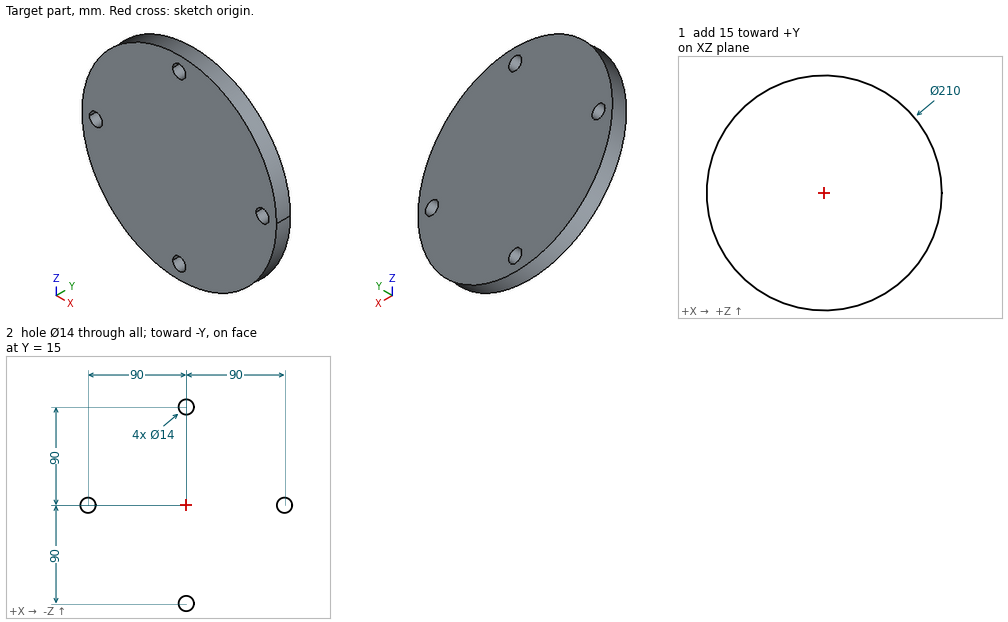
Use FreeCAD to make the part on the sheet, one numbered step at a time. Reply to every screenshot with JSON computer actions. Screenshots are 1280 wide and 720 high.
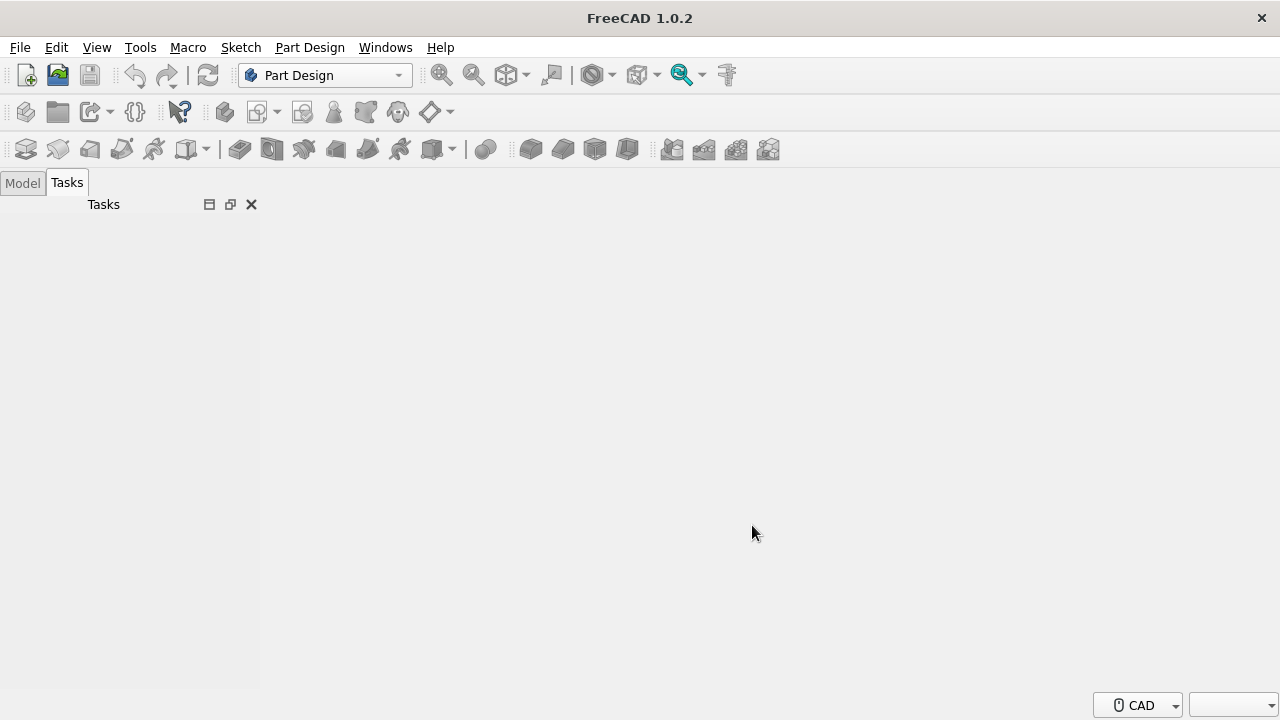
{"action": "key", "text": "ctrl+n"}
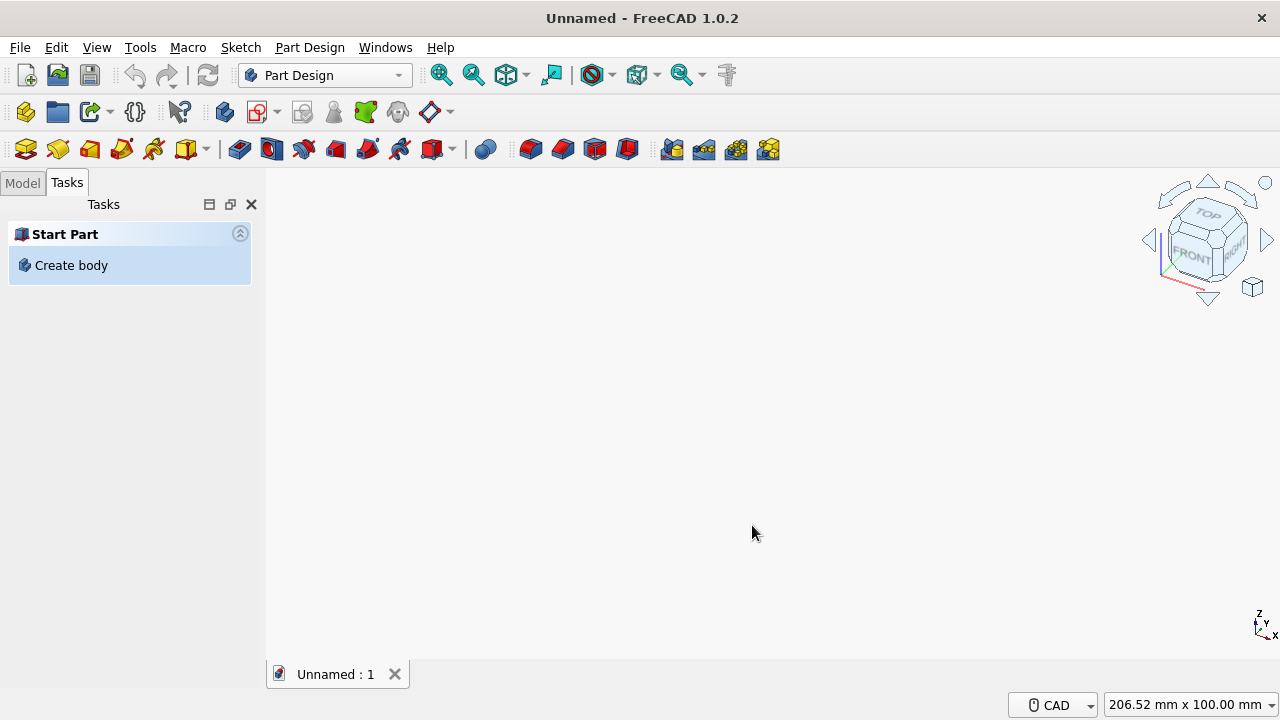
{"action": "left_click", "coordinate": [258, 112]}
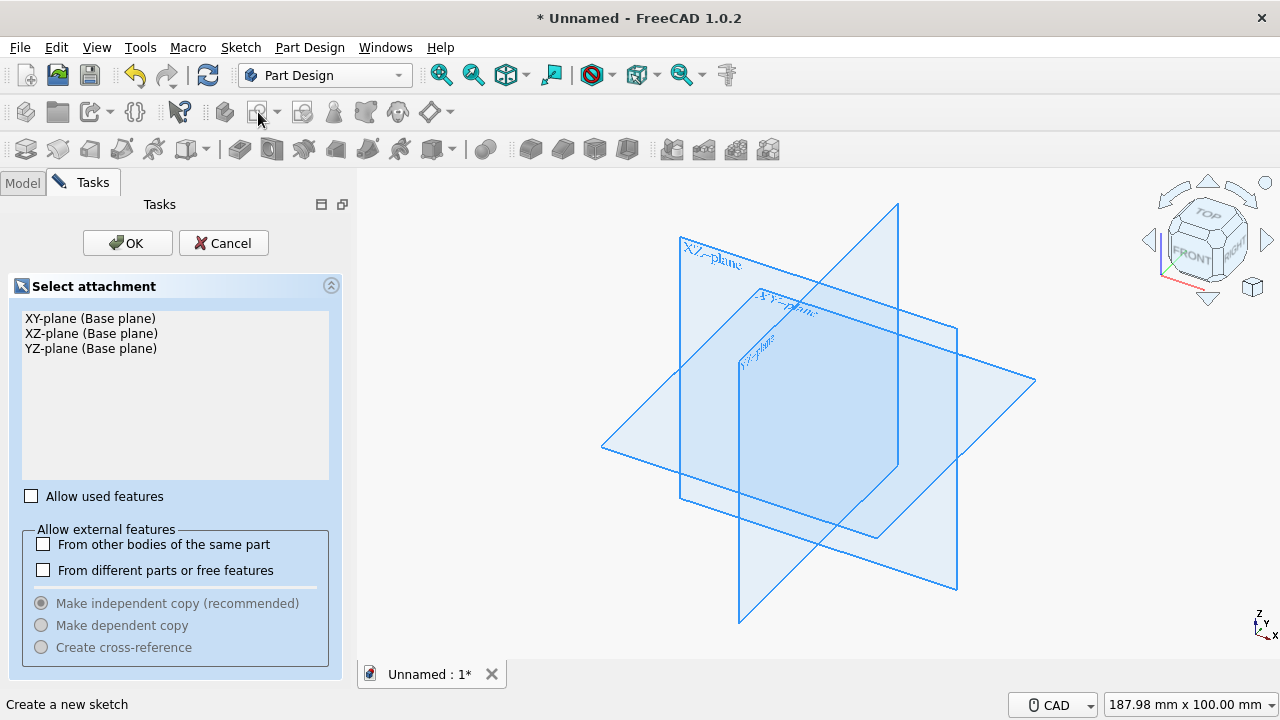
{"action": "left_click", "coordinate": [82, 334]}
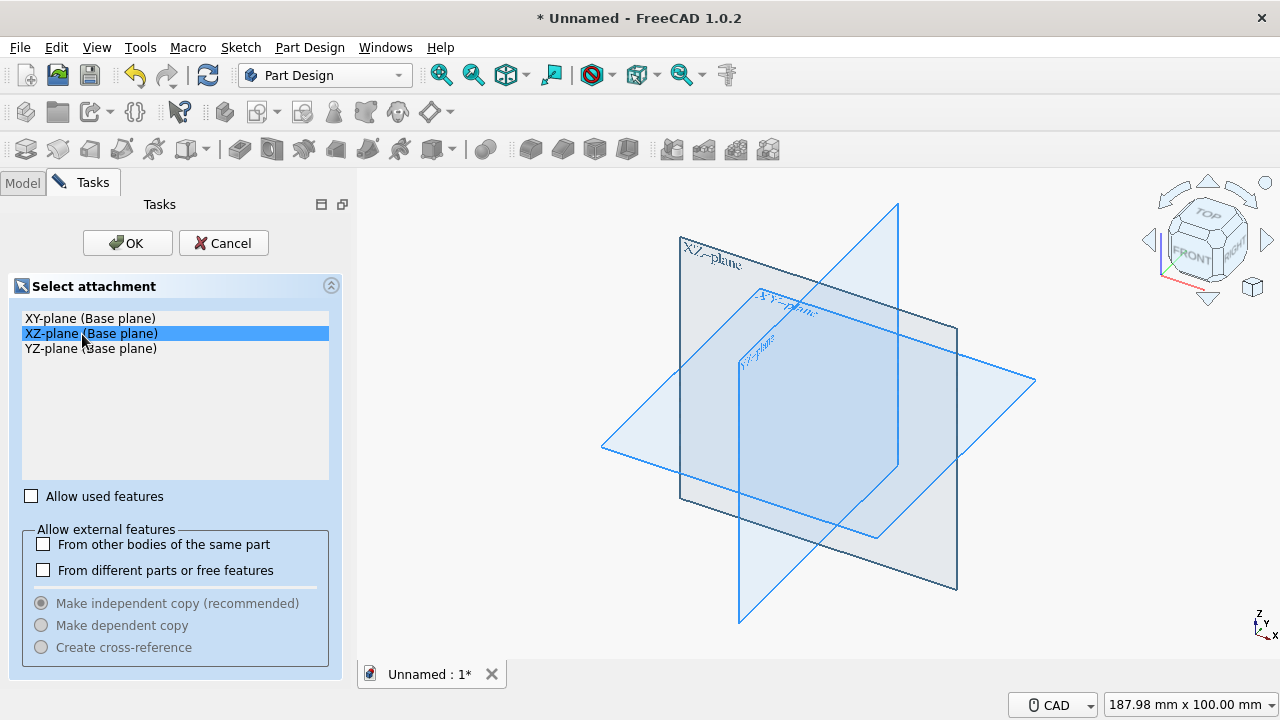
{"action": "left_click", "coordinate": [128, 243]}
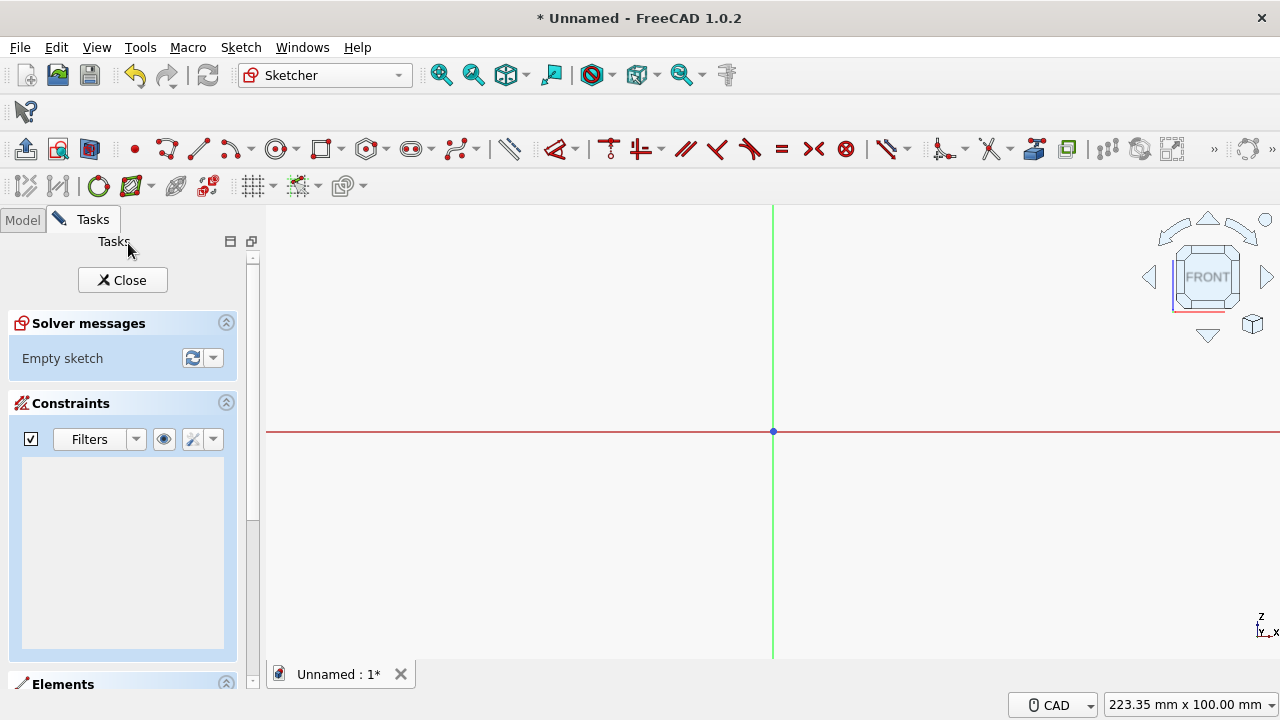
{"action": "scroll", "coordinate": [675, 432], "scroll_direction": "down", "scroll_amount": 6}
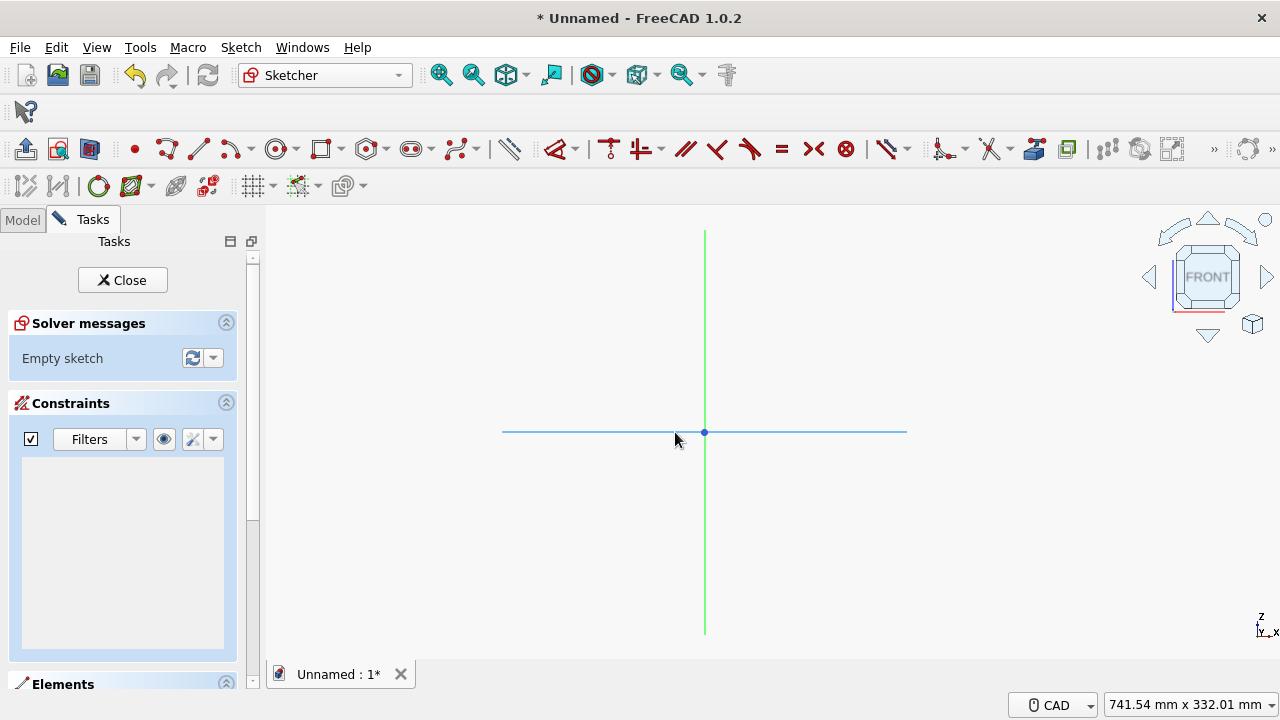
{"action": "left_click", "coordinate": [276, 150]}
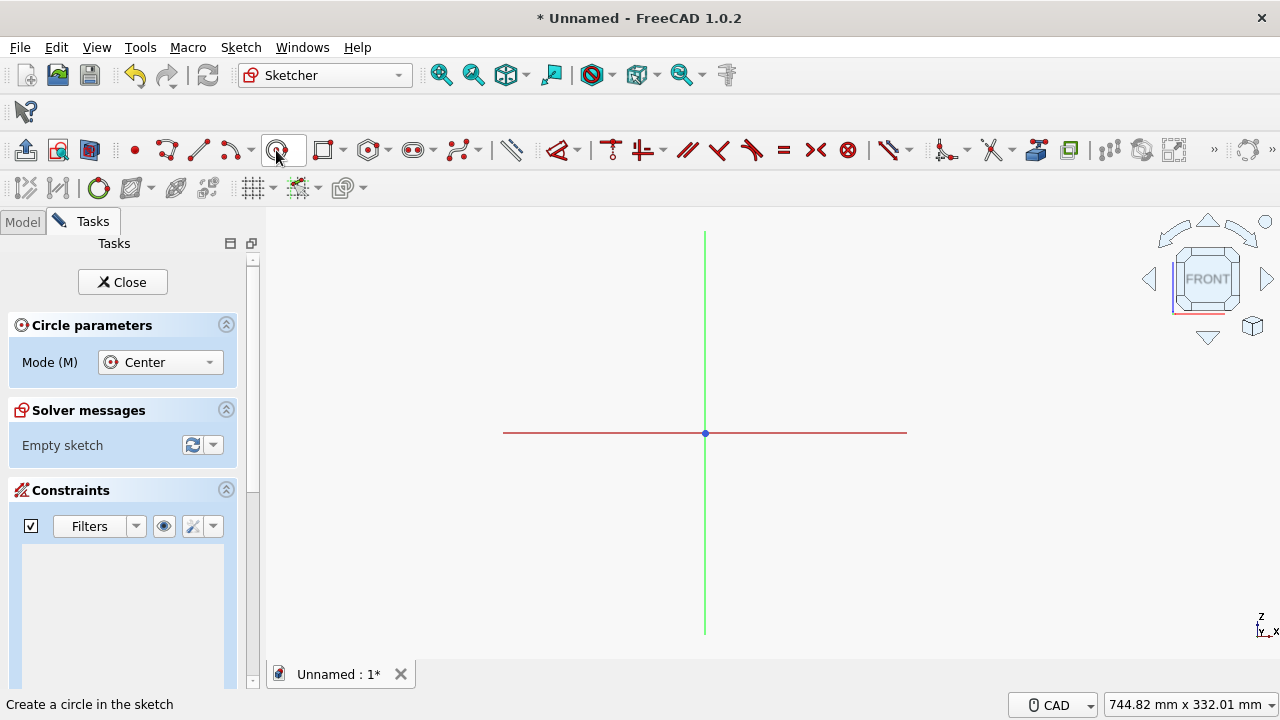
{"action": "left_click", "coordinate": [705, 433]}
{"action": "mouse_move", "coordinate": [806, 332]}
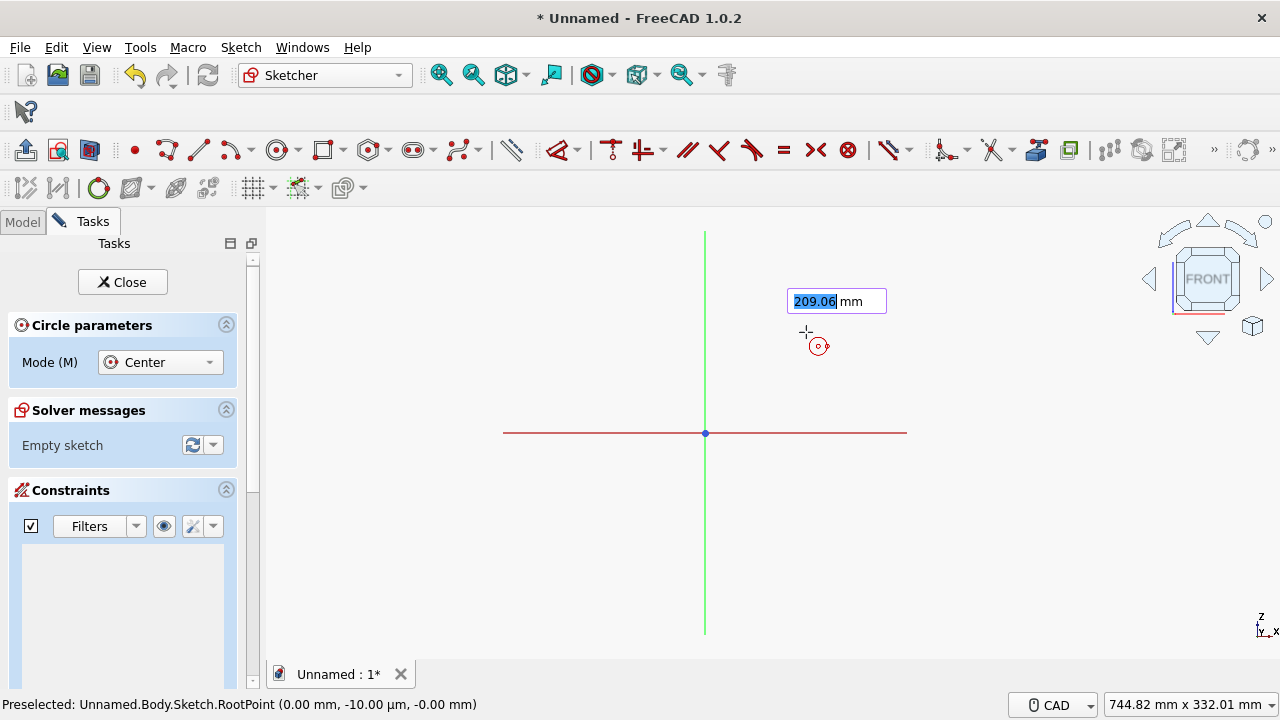
{"action": "type", "text": "210"}
{"action": "key", "text": "Return"}
{"action": "key", "text": "Escape"}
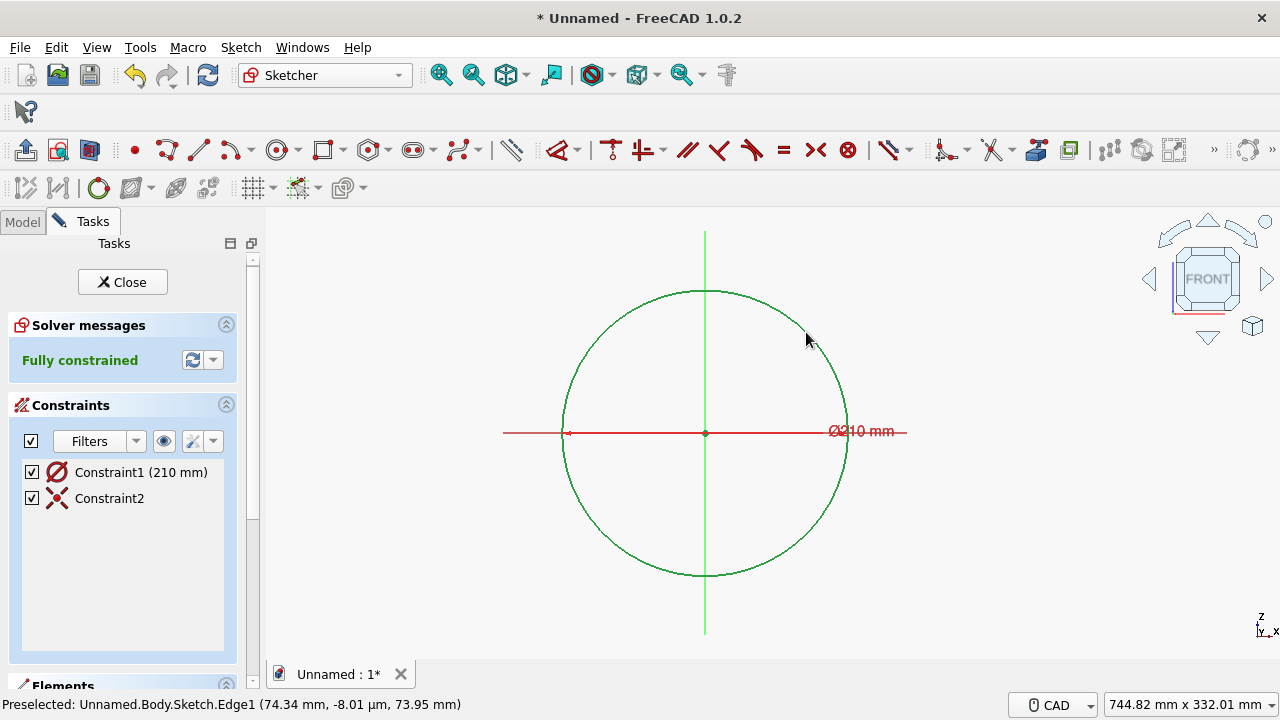
{"action": "left_click", "coordinate": [123, 282]}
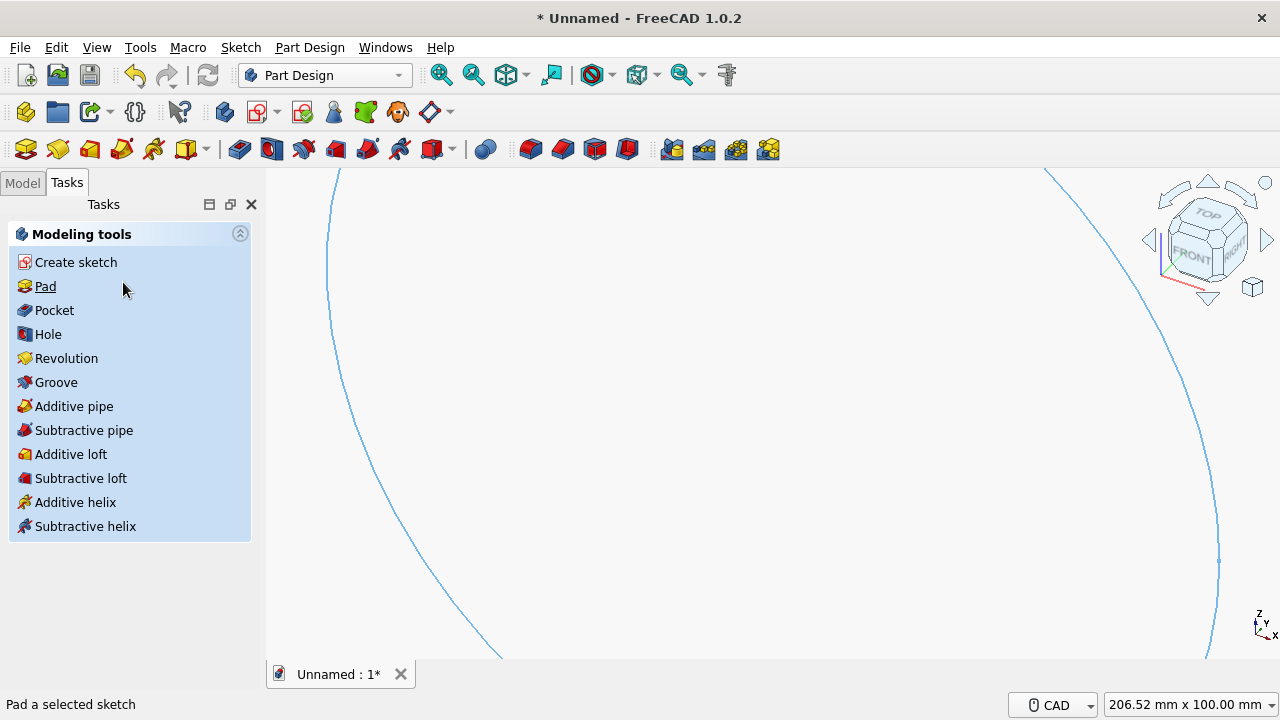
{"action": "left_click", "coordinate": [26, 150]}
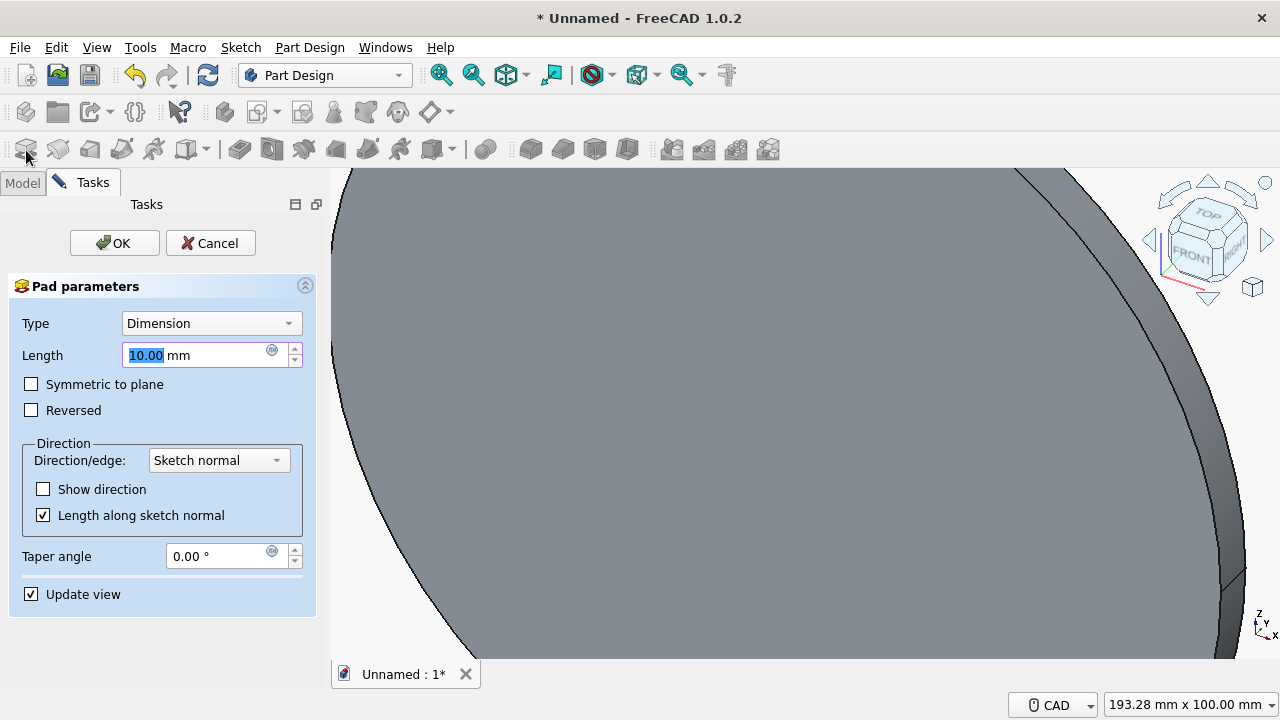
{"action": "type", "text": "15"}
{"action": "key", "text": "Tab"}